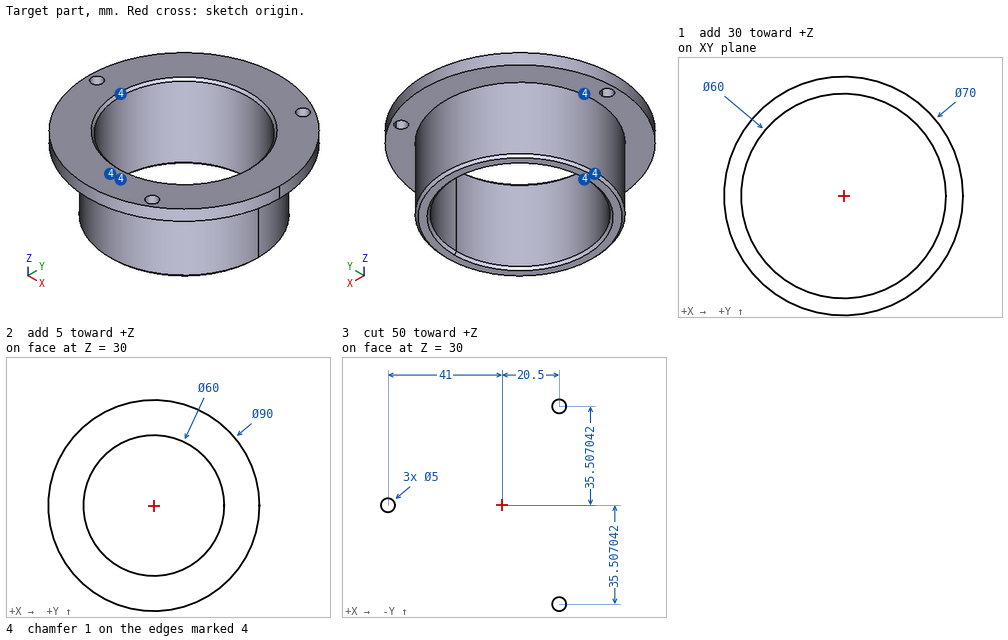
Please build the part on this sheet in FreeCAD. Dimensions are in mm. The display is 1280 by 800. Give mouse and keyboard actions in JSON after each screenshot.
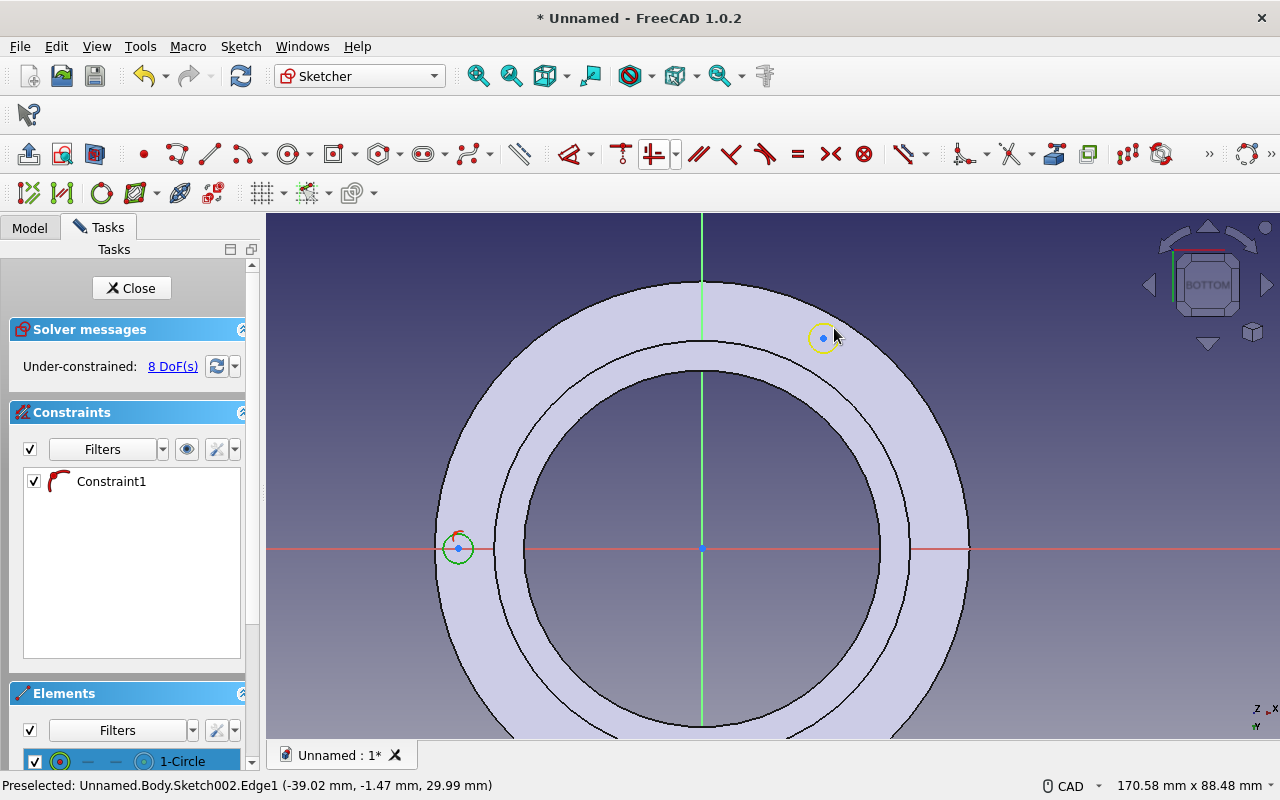
{"action": "left_click", "coordinate": [834, 328]}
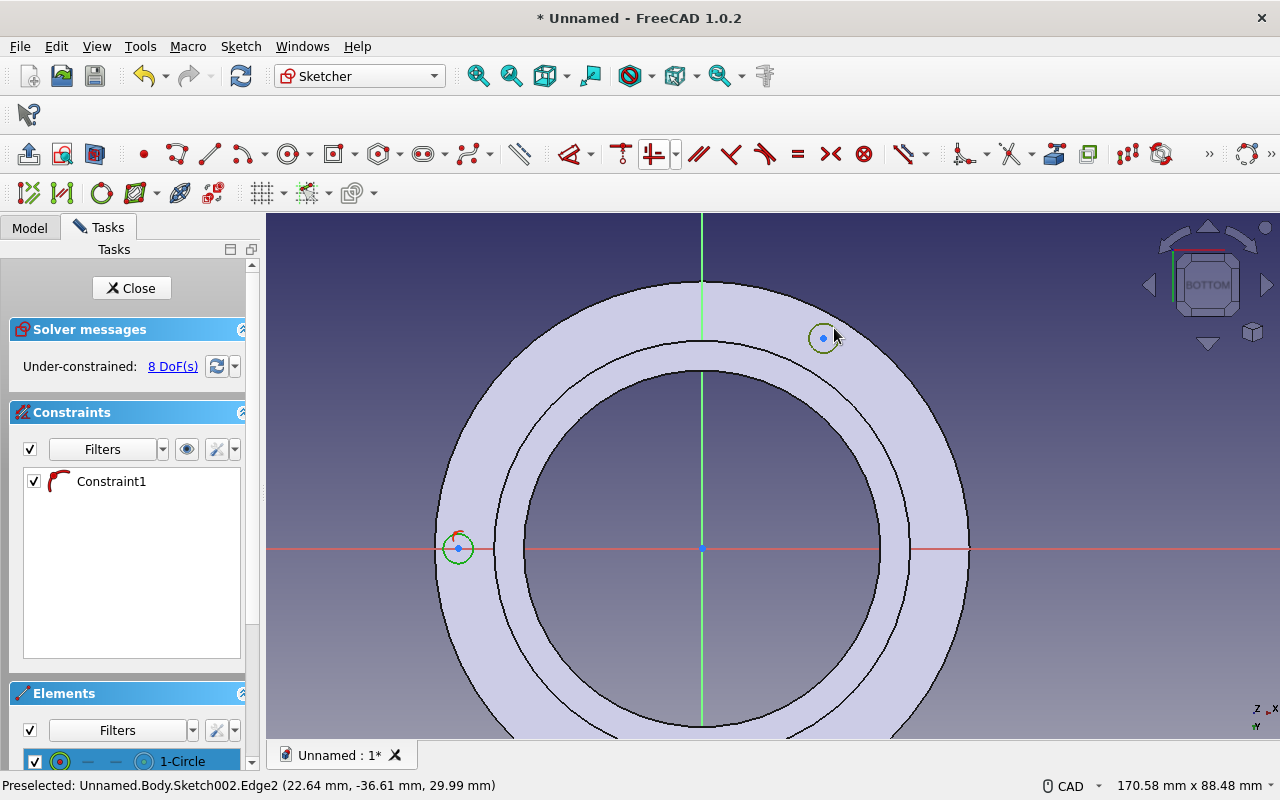
{"action": "scroll", "coordinate": [833, 328], "scroll_direction": "down", "scroll_amount": 2}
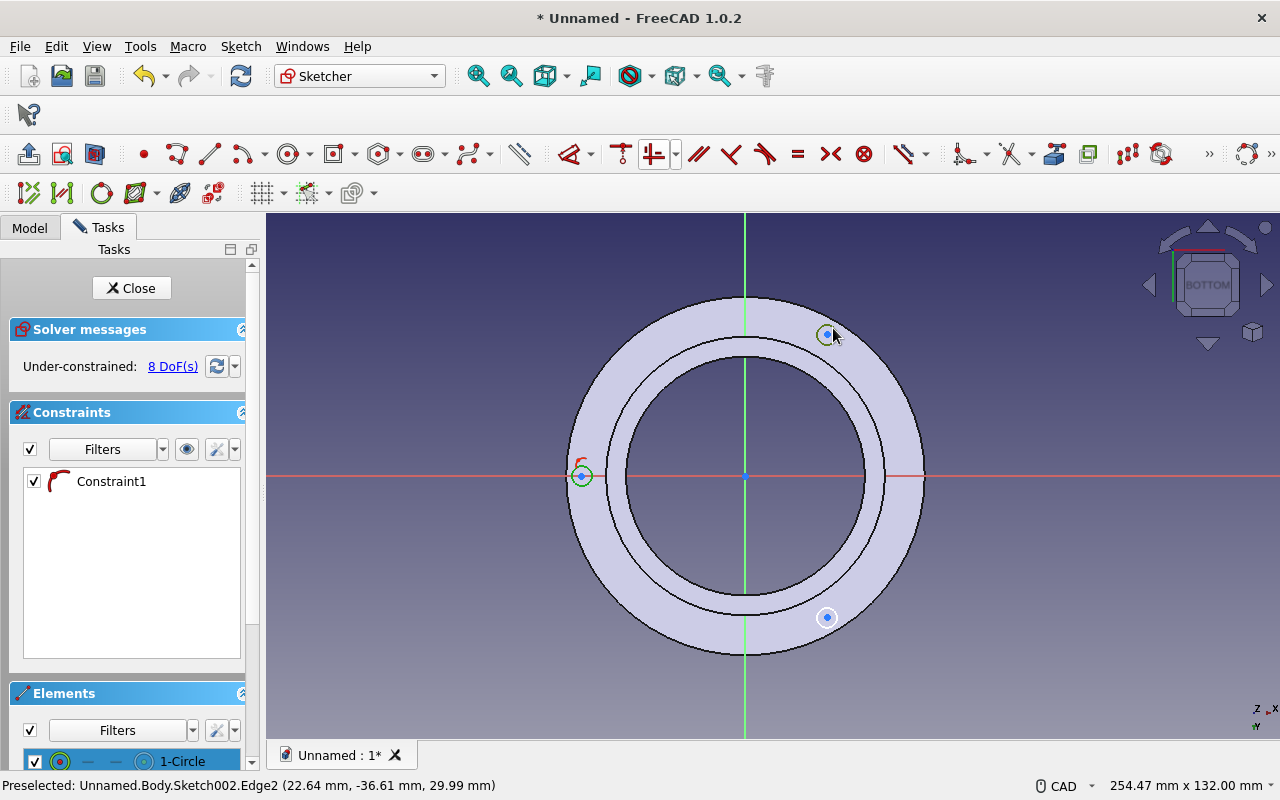
{"action": "scroll", "coordinate": [834, 611], "scroll_direction": "up", "scroll_amount": 2}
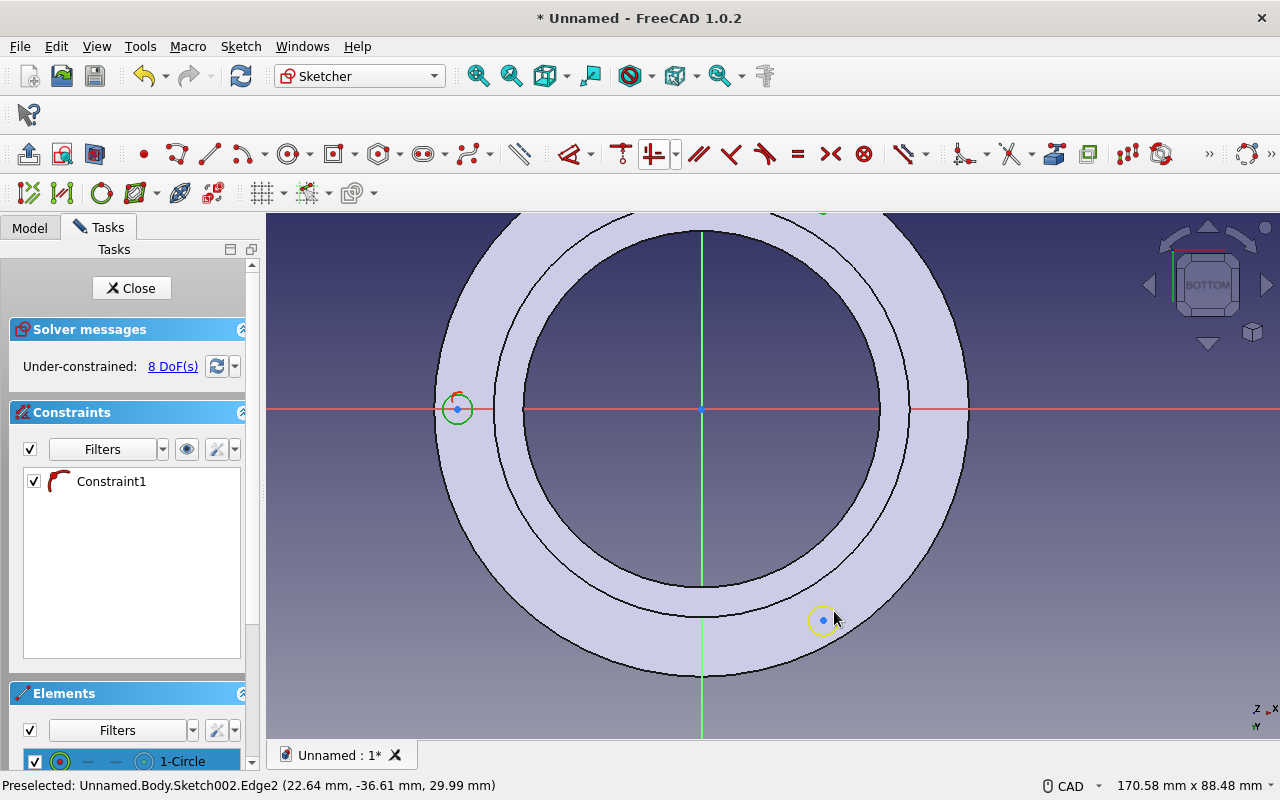
{"action": "left_click", "coordinate": [834, 611]}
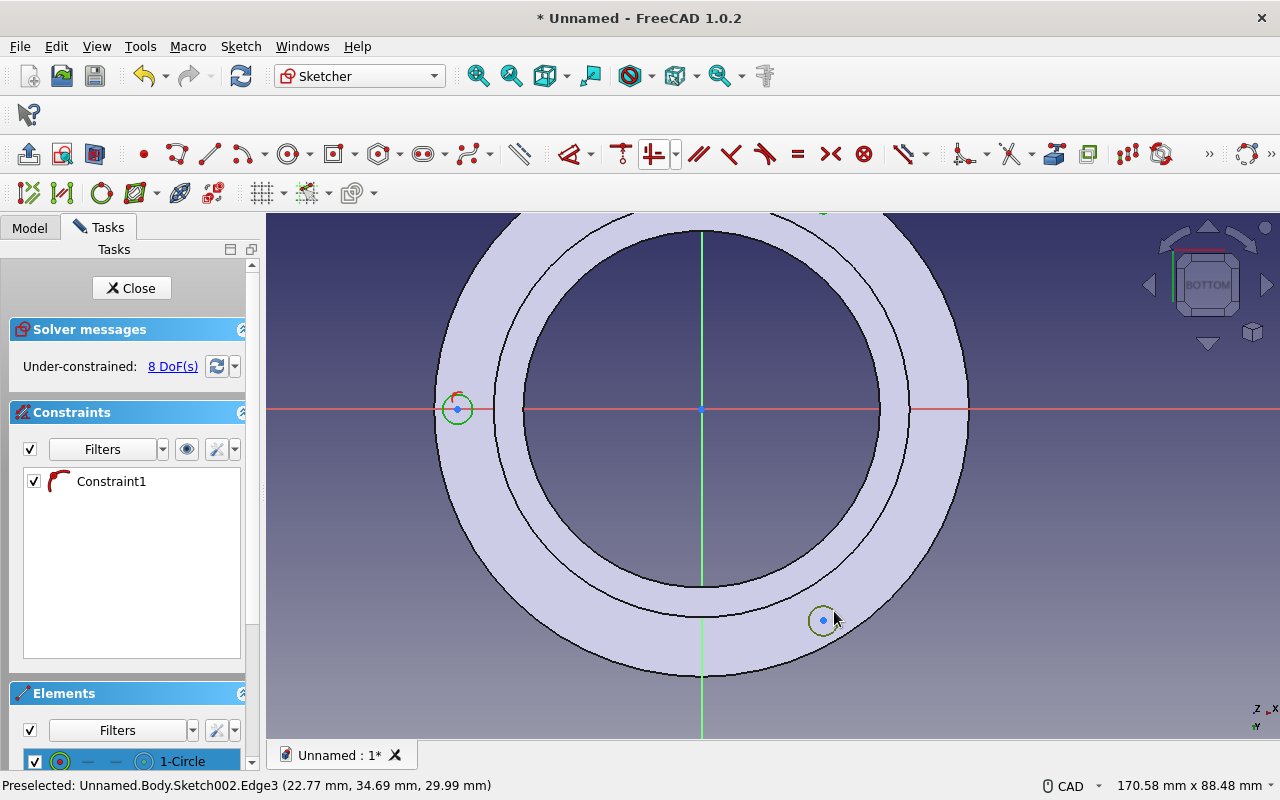
{"action": "left_click", "coordinate": [798, 154]}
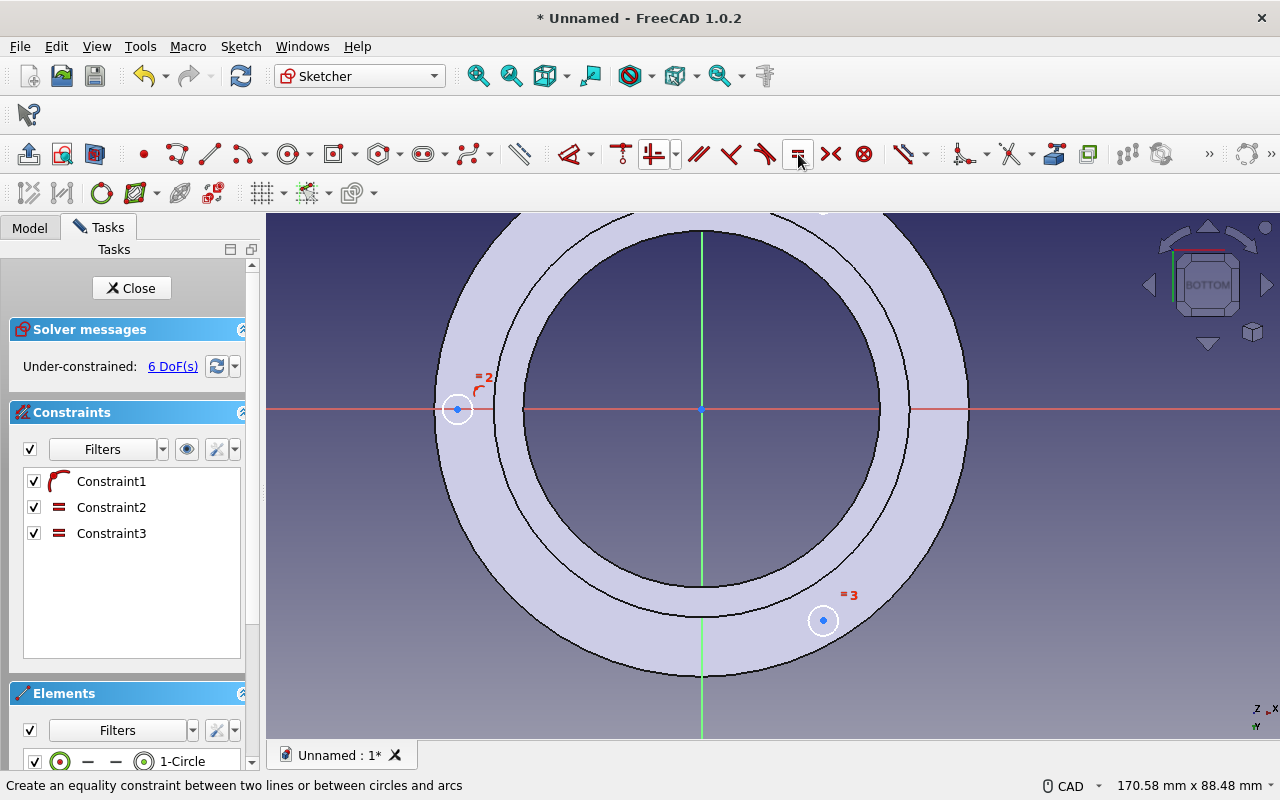
{"action": "scroll", "coordinate": [834, 612], "scroll_direction": "down", "scroll_amount": 2}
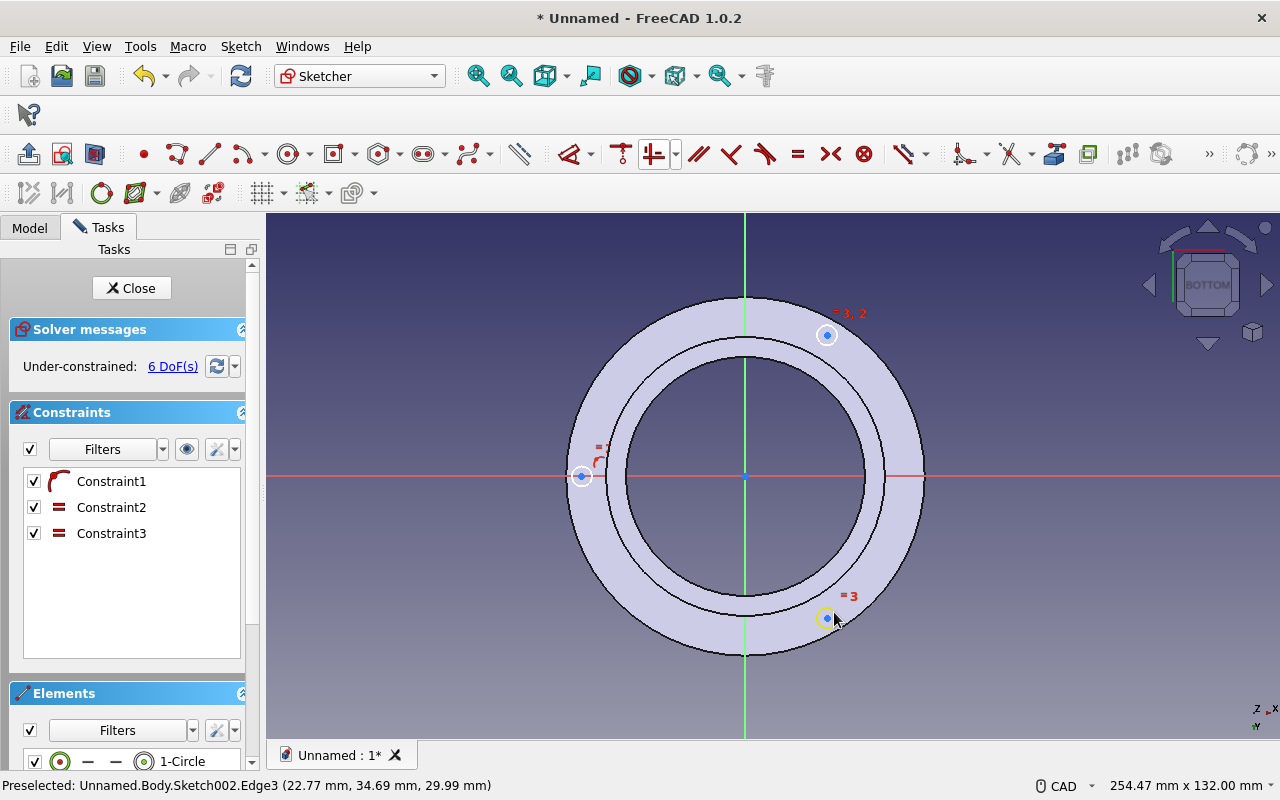
{"action": "left_click", "coordinate": [827, 335]}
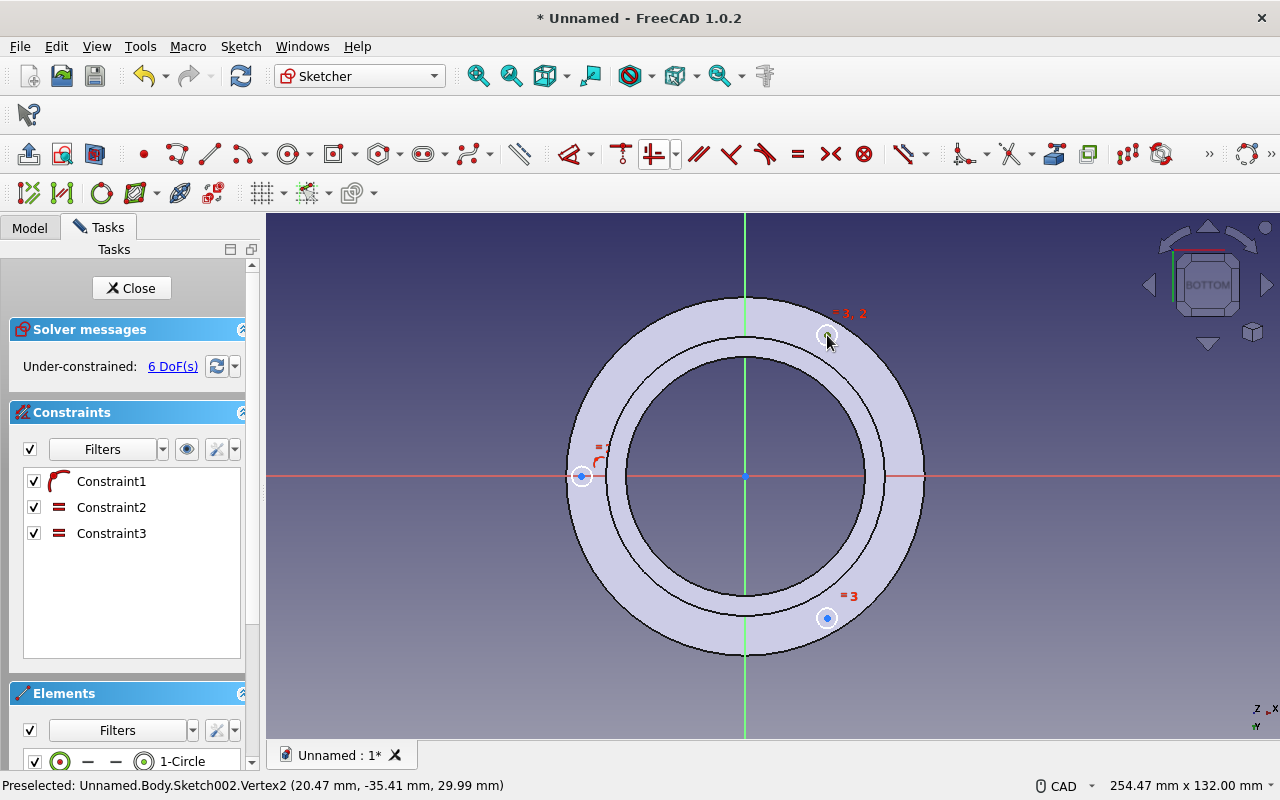
{"action": "left_click", "coordinate": [827, 618]}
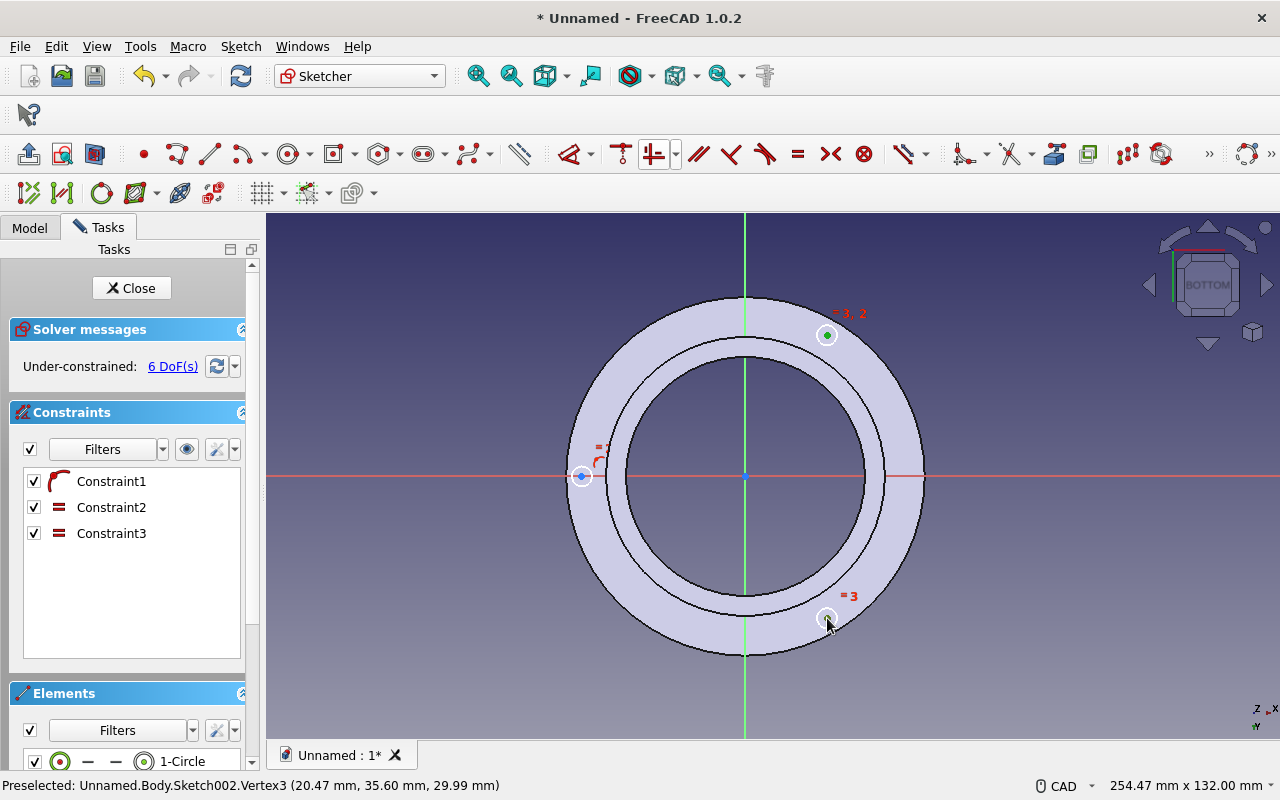
{"action": "key", "text": "v"}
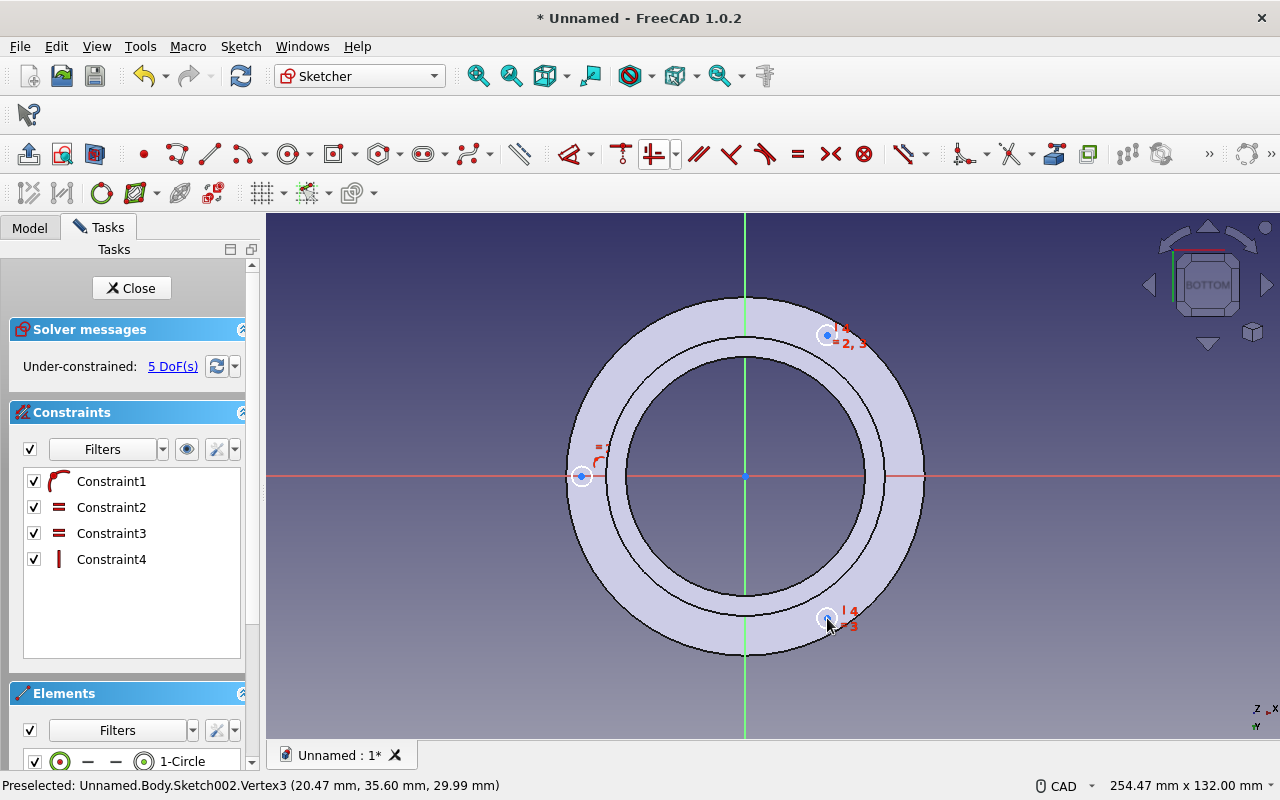
{"action": "left_click", "coordinate": [568, 154]}